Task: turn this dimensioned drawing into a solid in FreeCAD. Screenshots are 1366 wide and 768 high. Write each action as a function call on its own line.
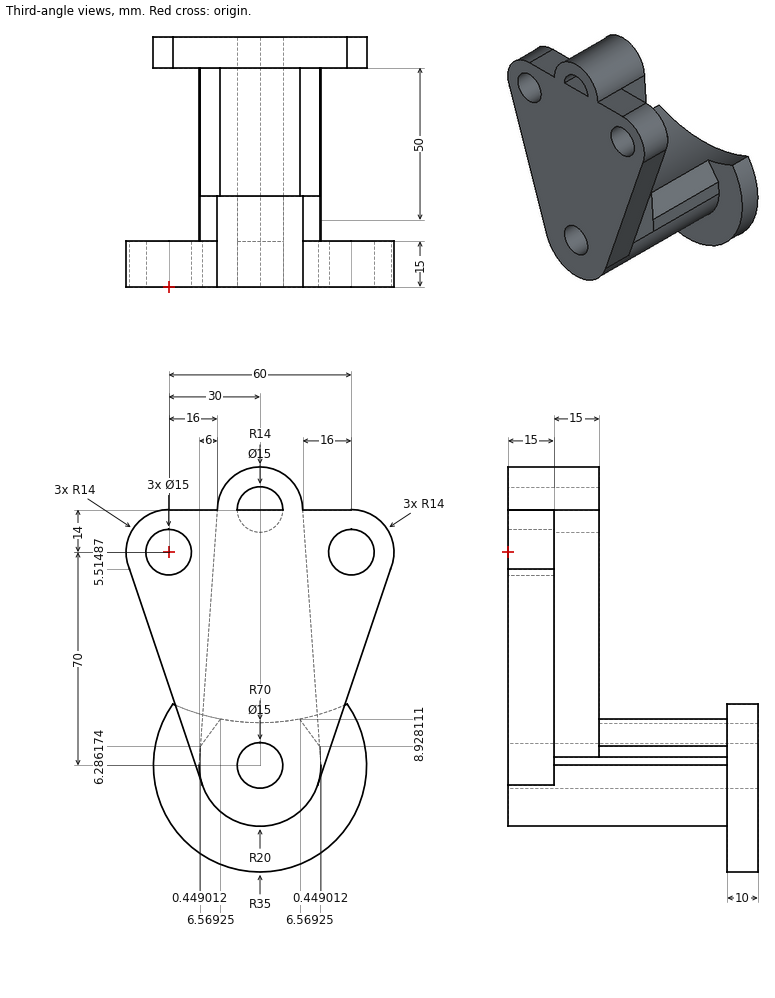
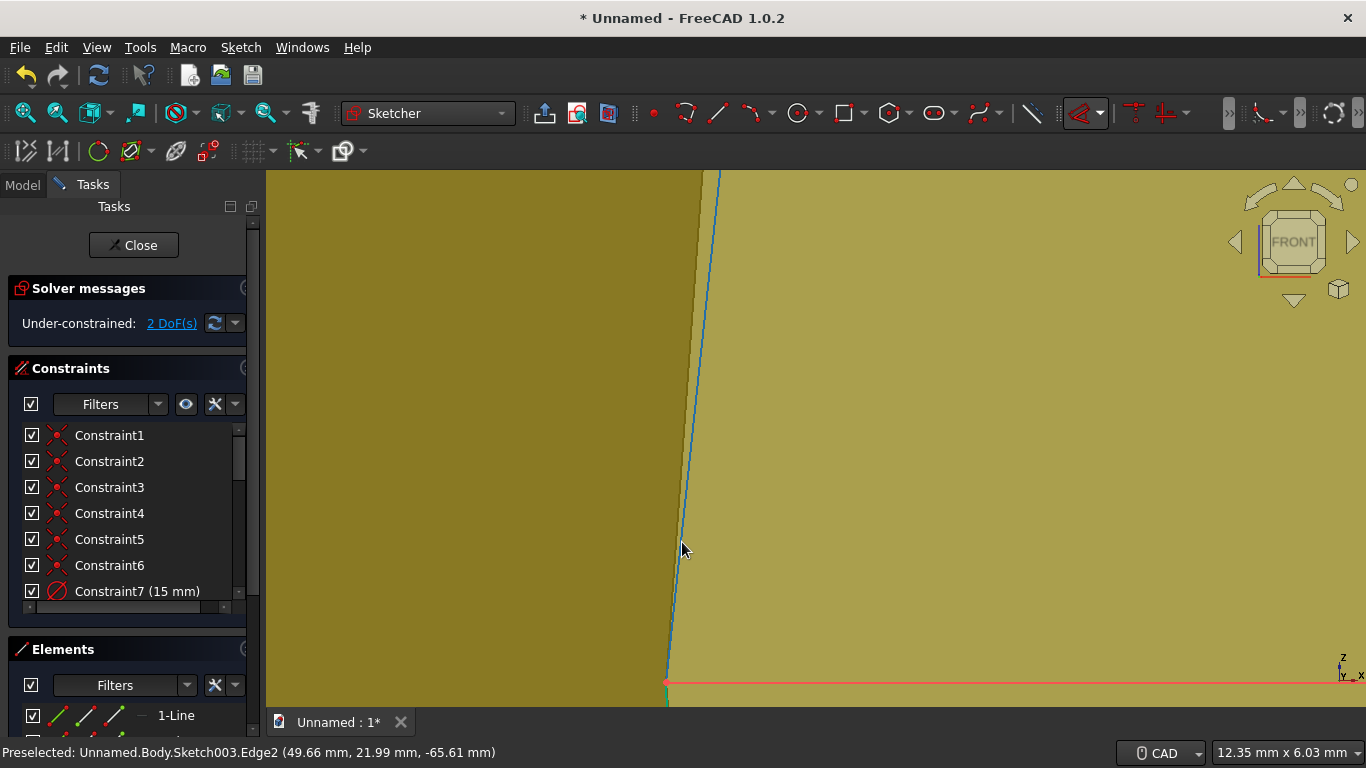
click(683, 519)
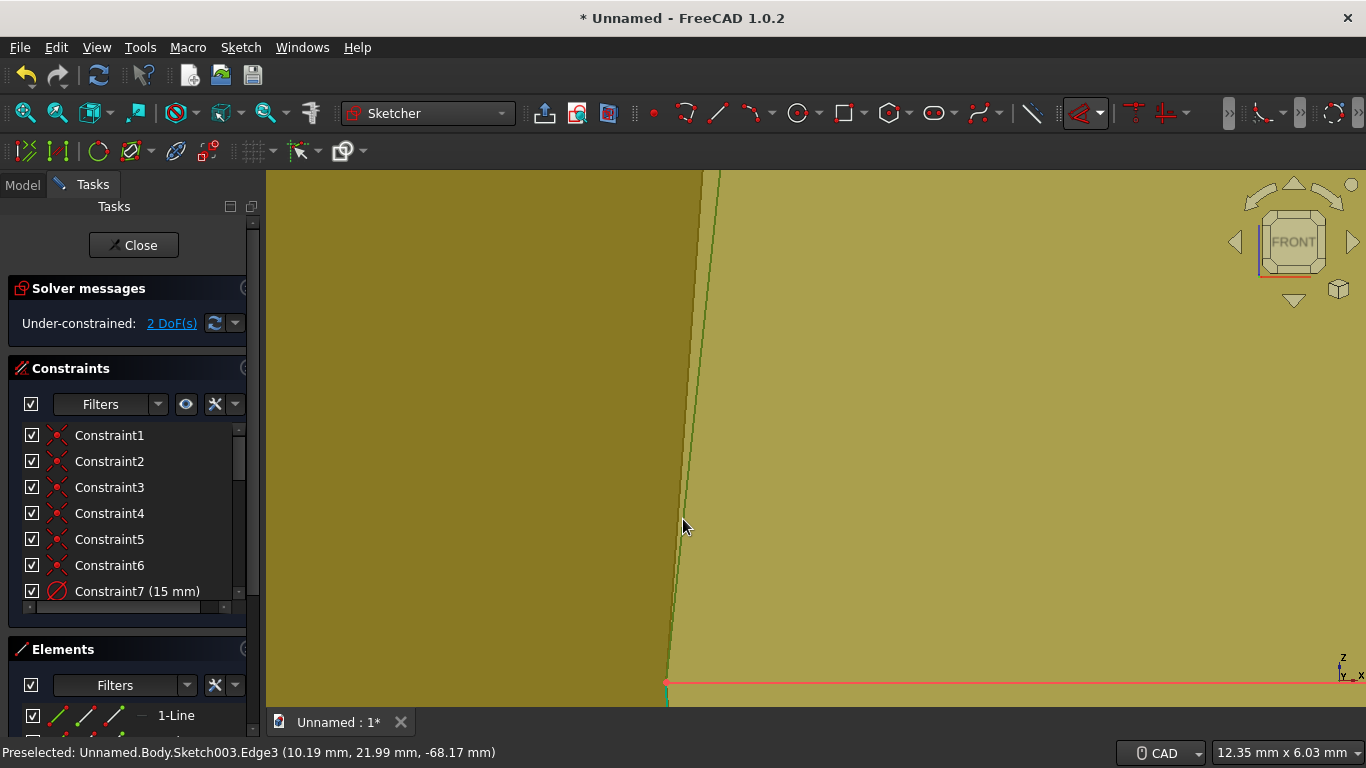
click(1102, 114)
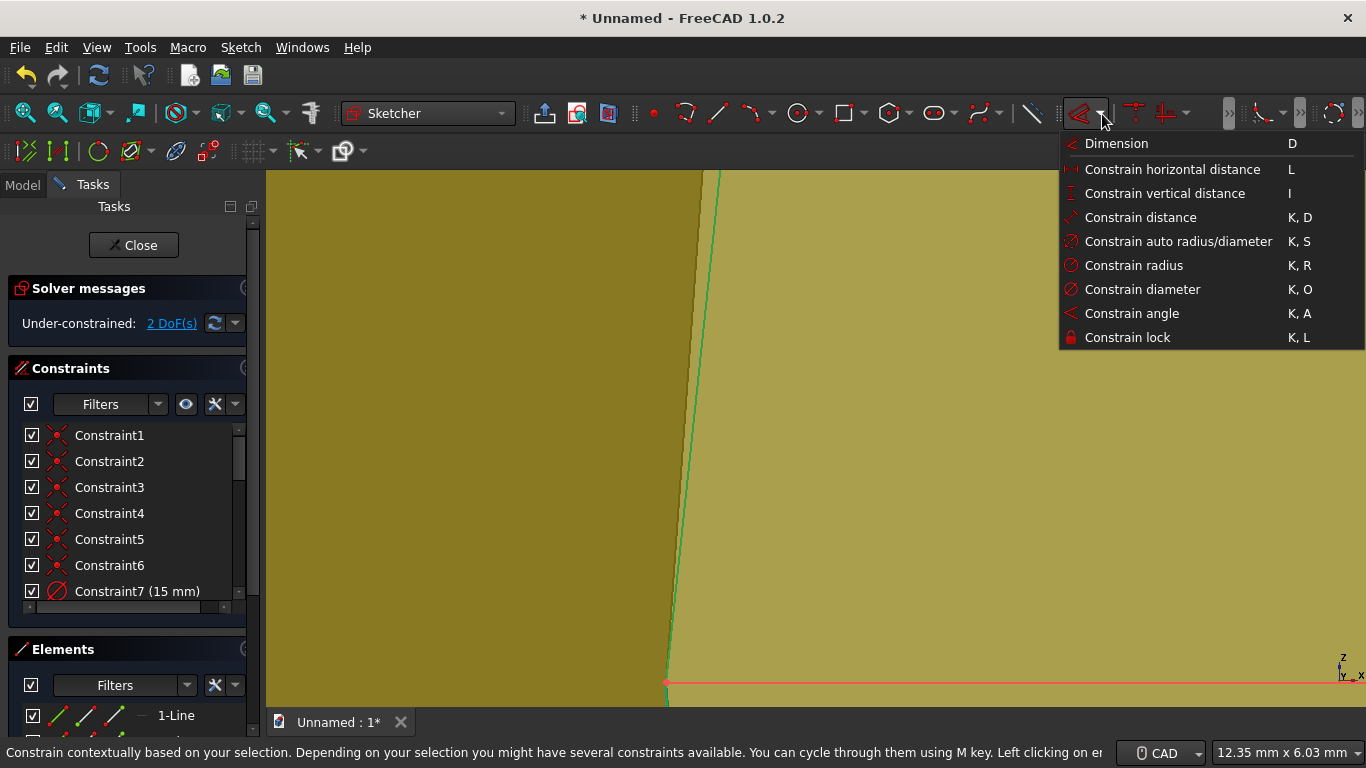
click(1212, 169)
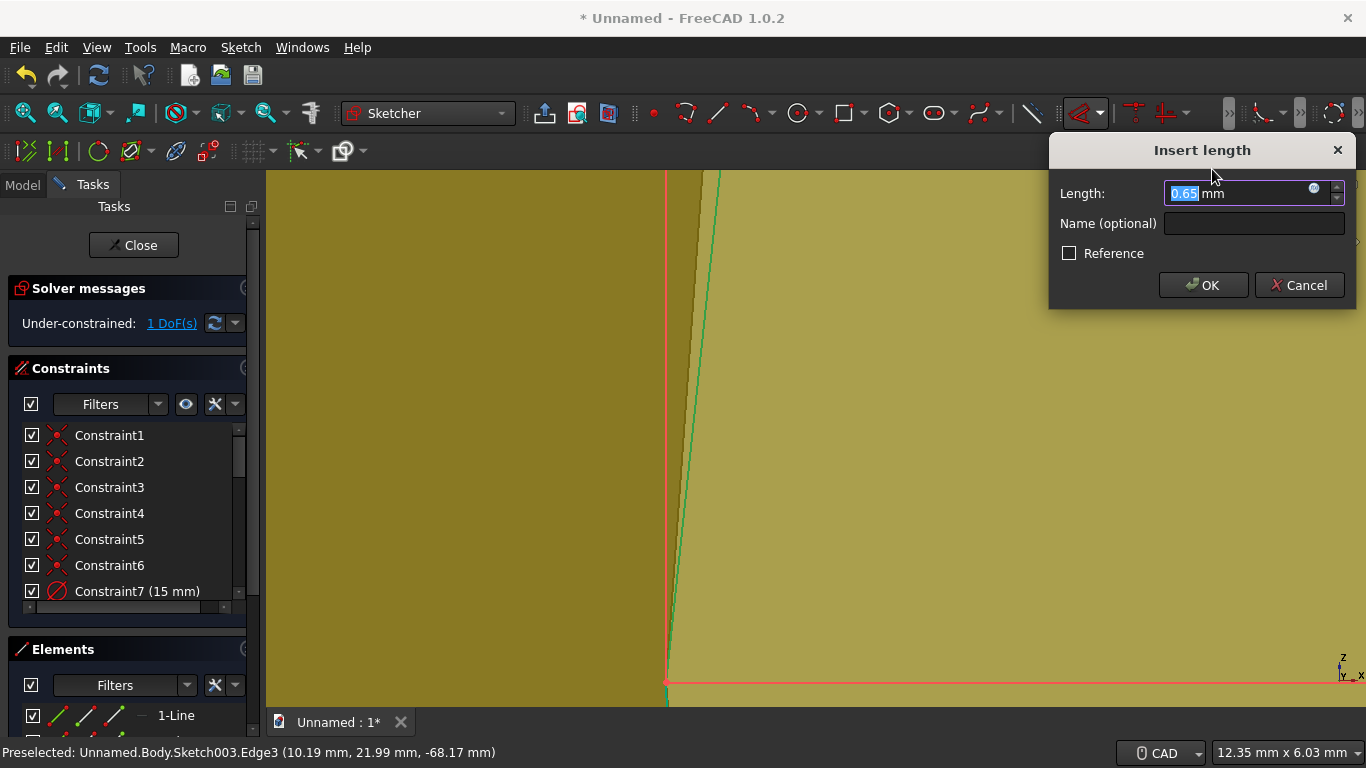
text(0.449012)
key(Return)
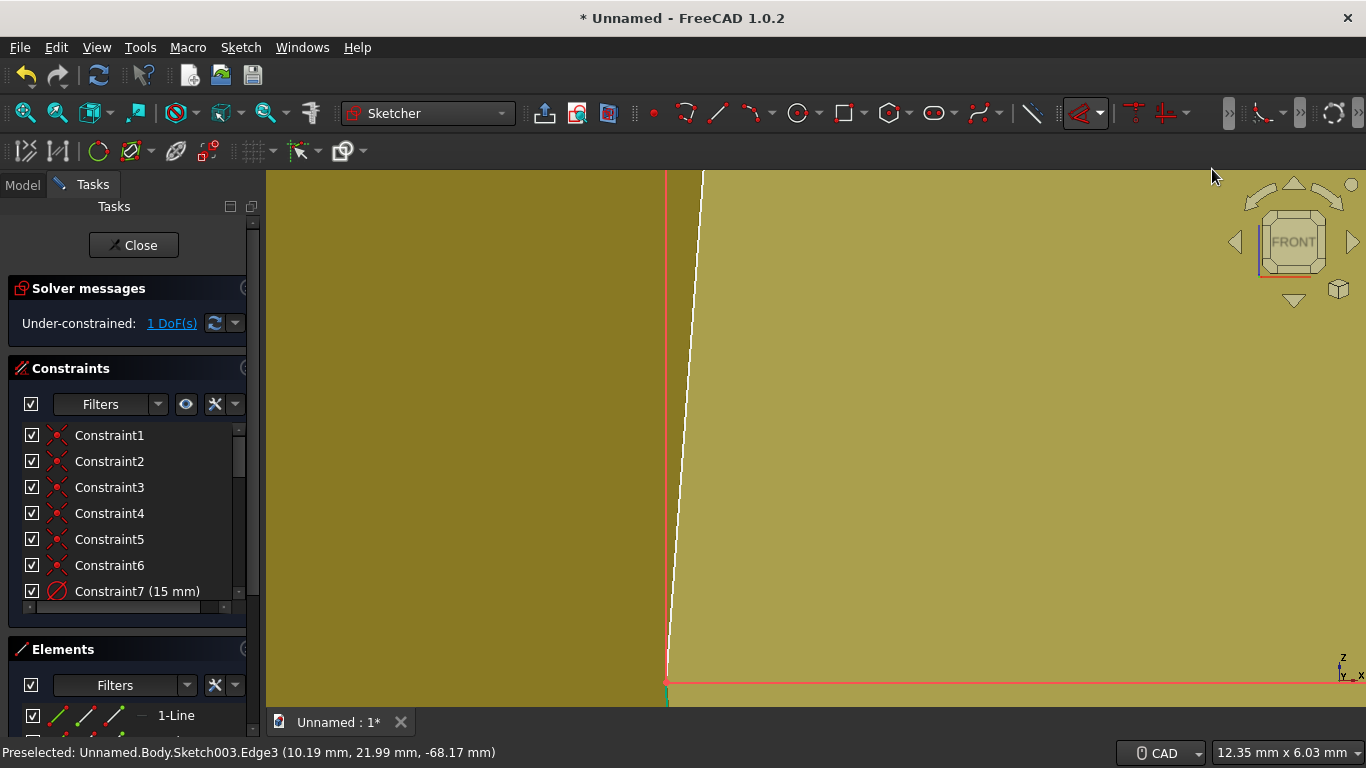
scroll(682, 542, down, 15)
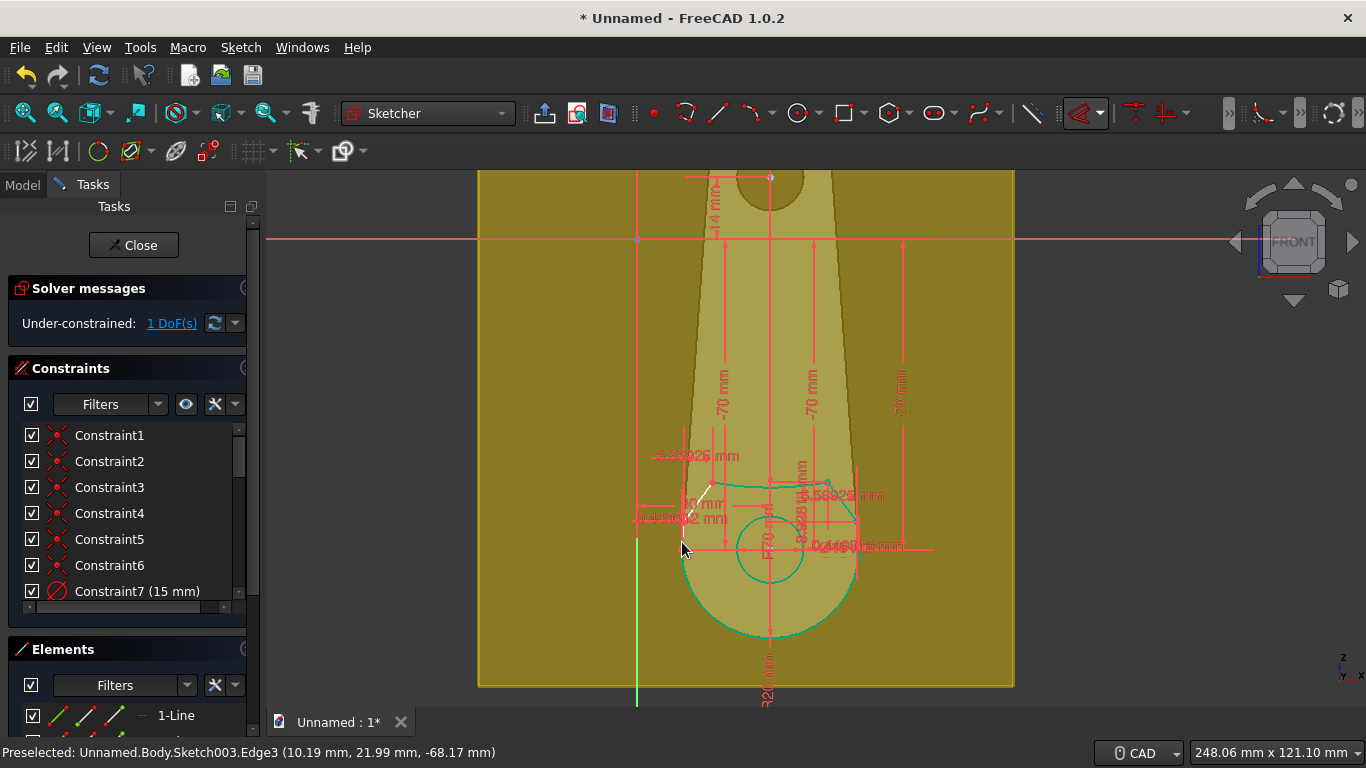
scroll(682, 542, up, 3)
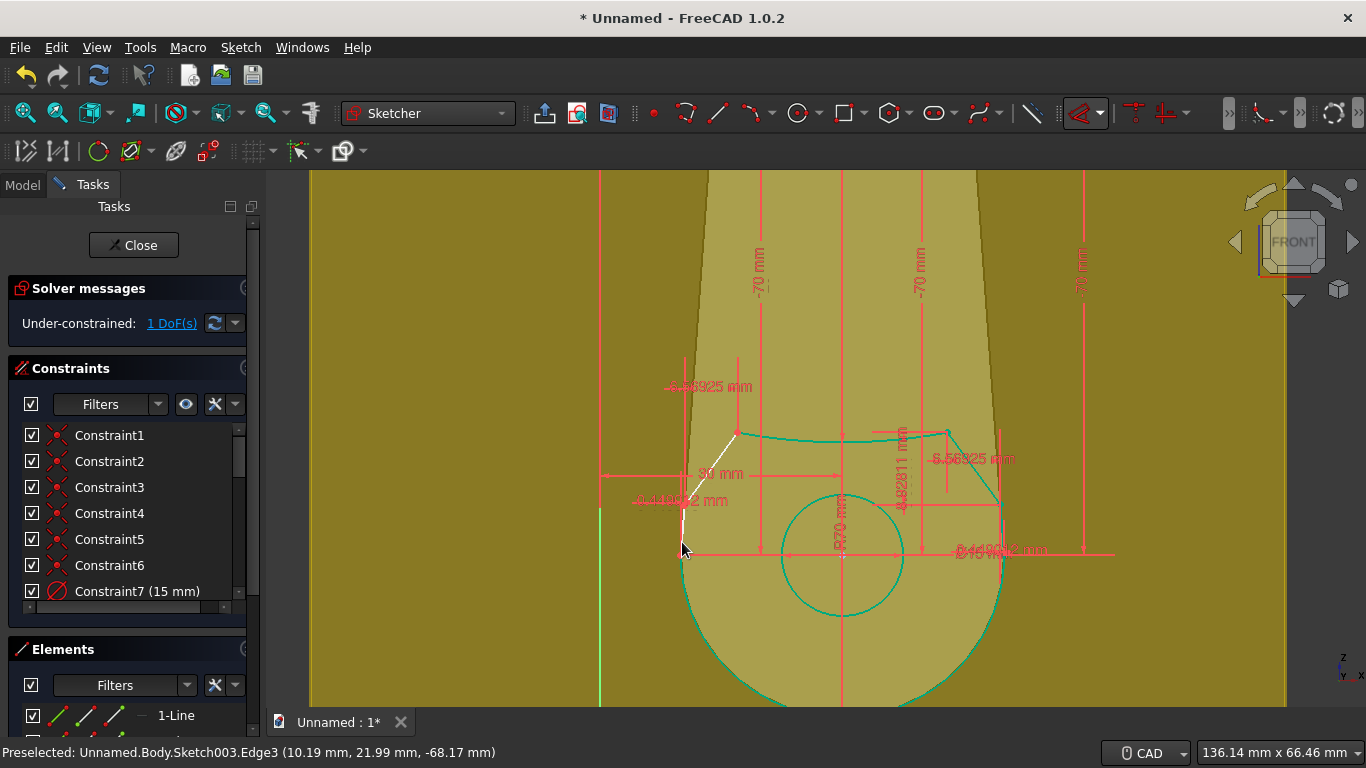
click(682, 541)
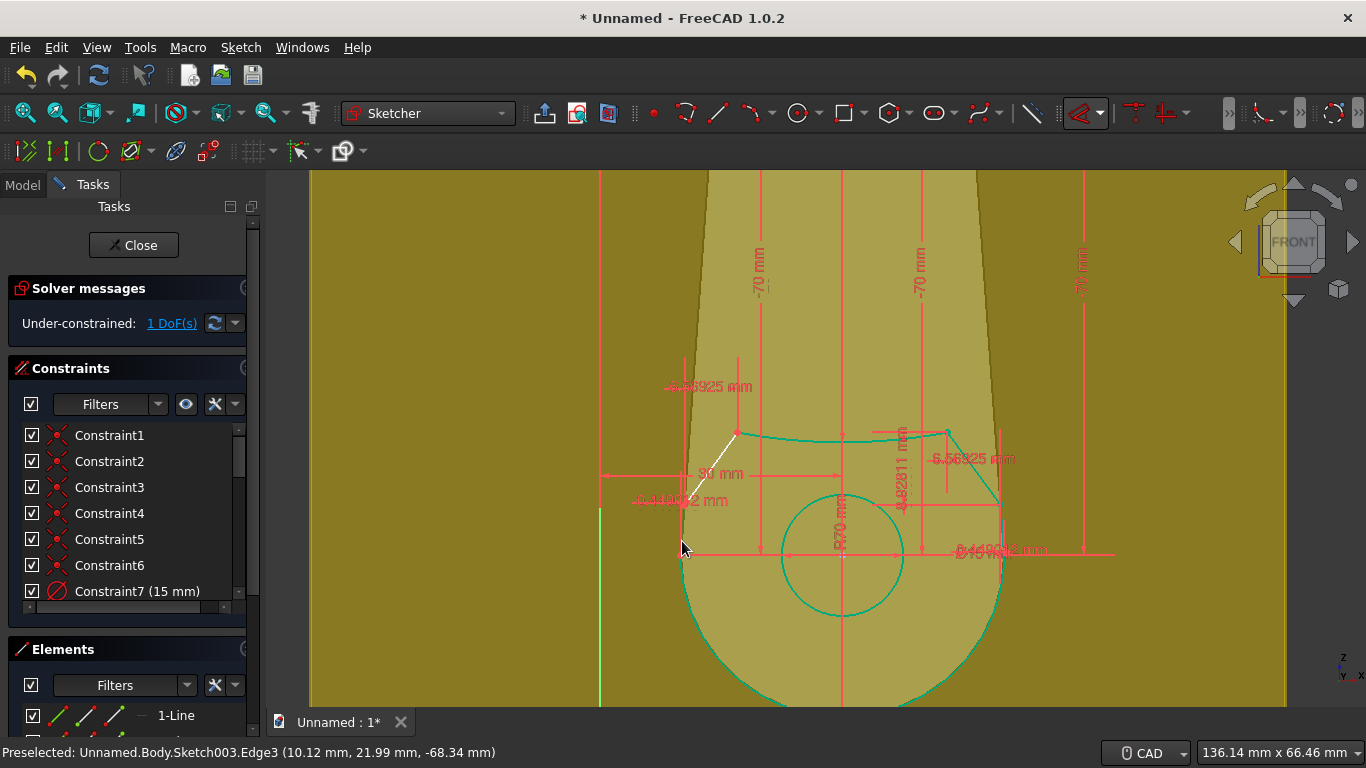
click(1102, 114)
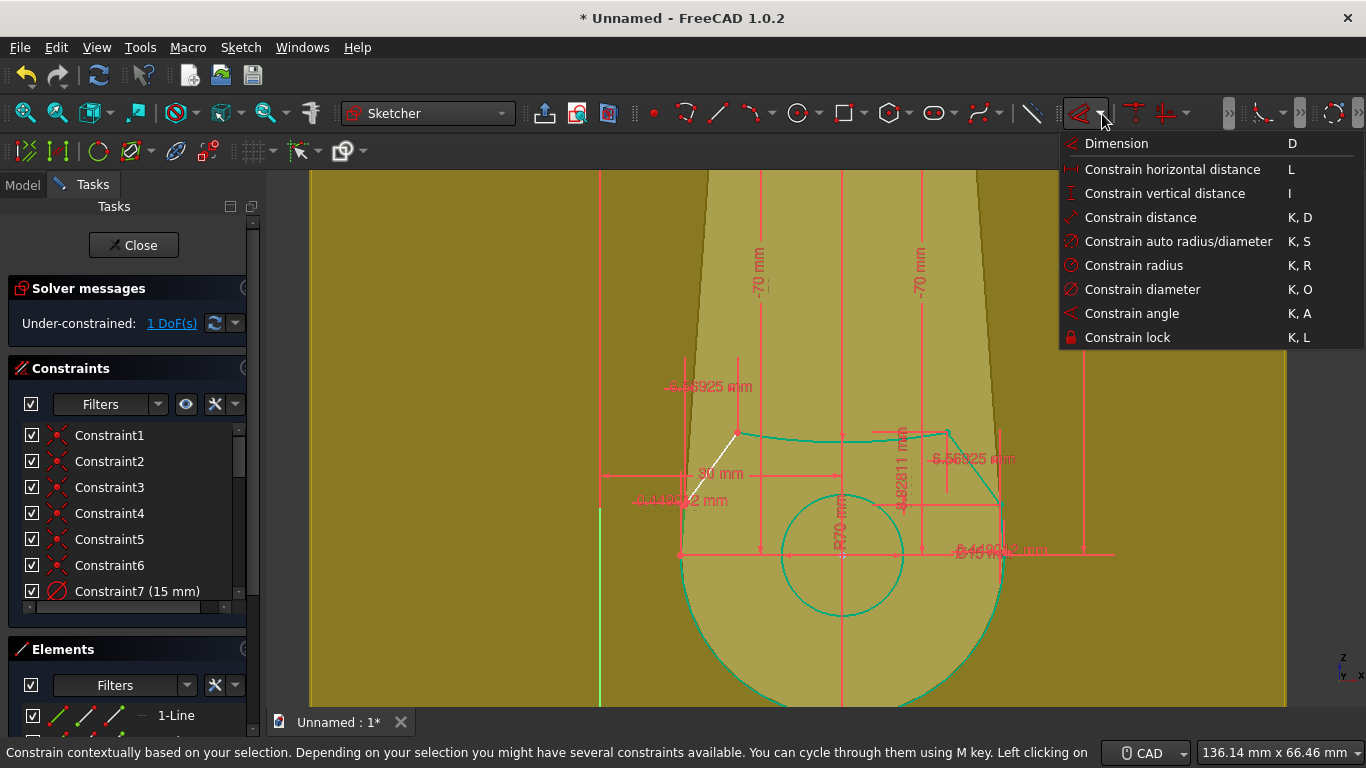
click(1212, 193)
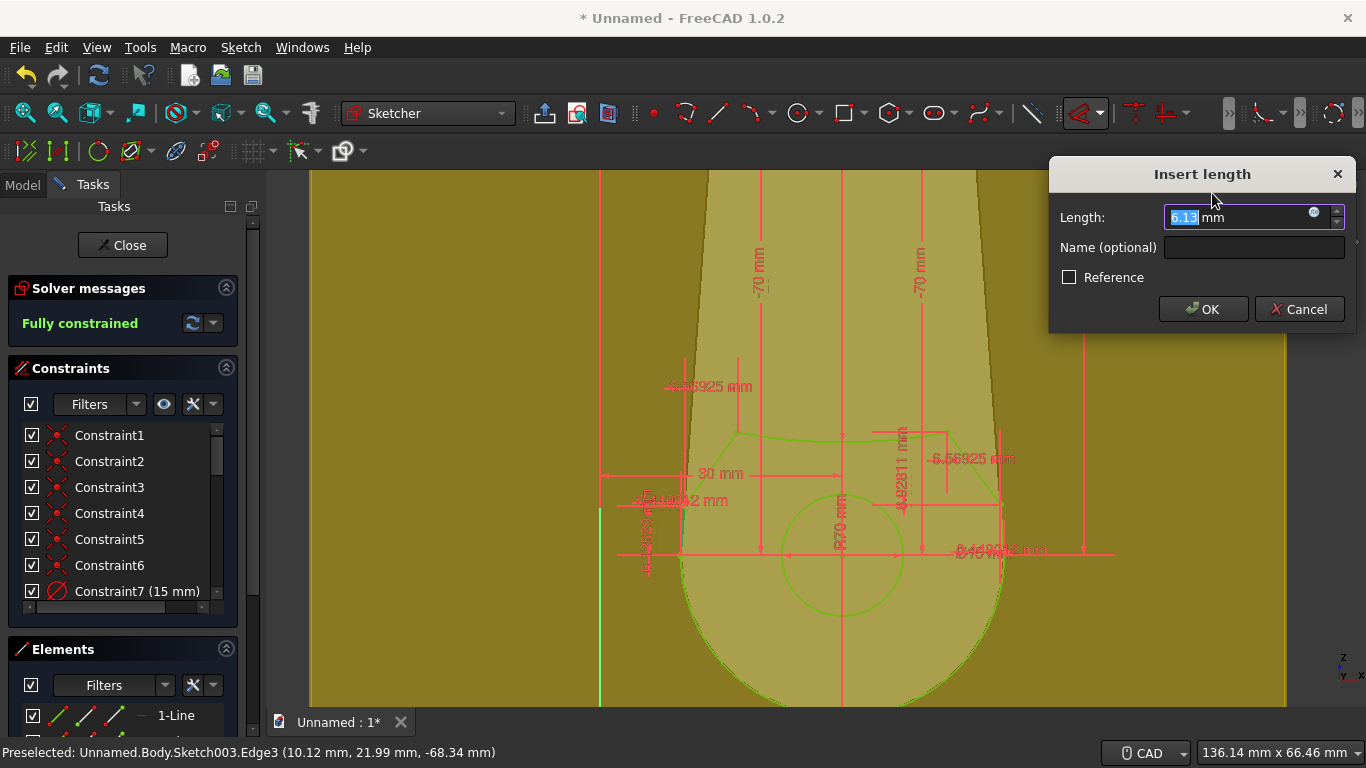
text(6.286174)
key(Return)